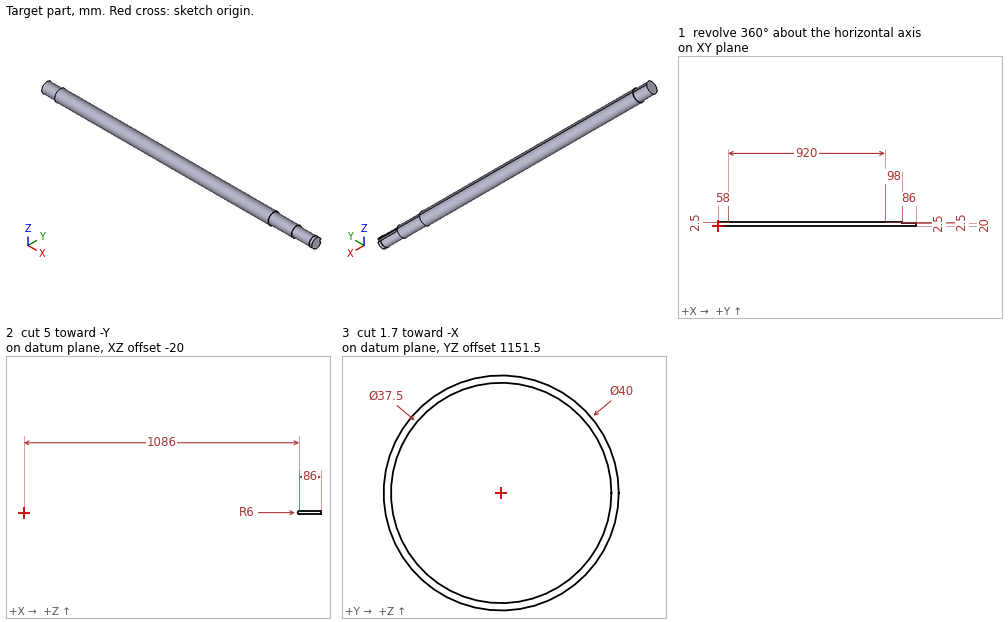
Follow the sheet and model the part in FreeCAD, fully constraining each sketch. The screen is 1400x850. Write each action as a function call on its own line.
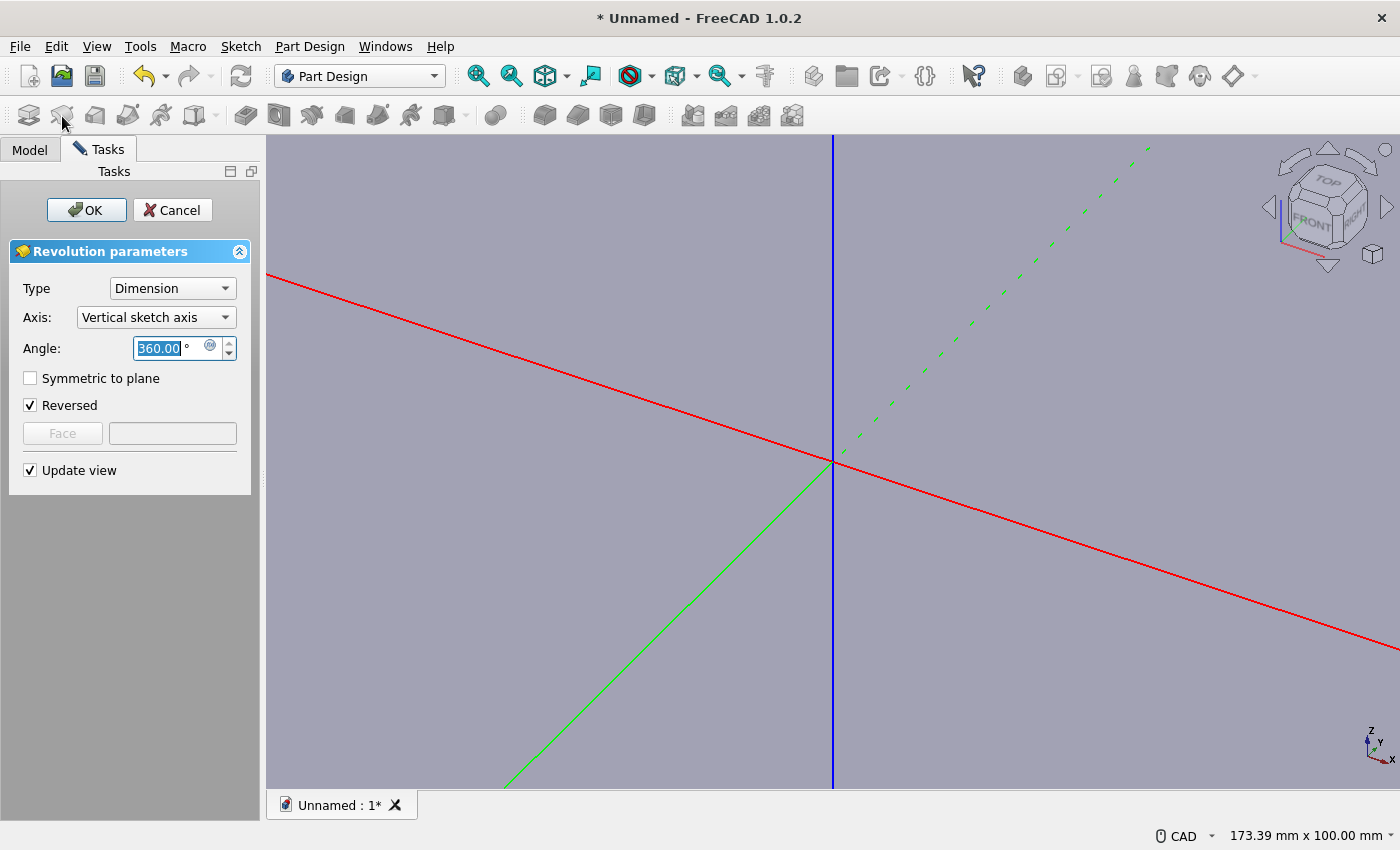
click(157, 318)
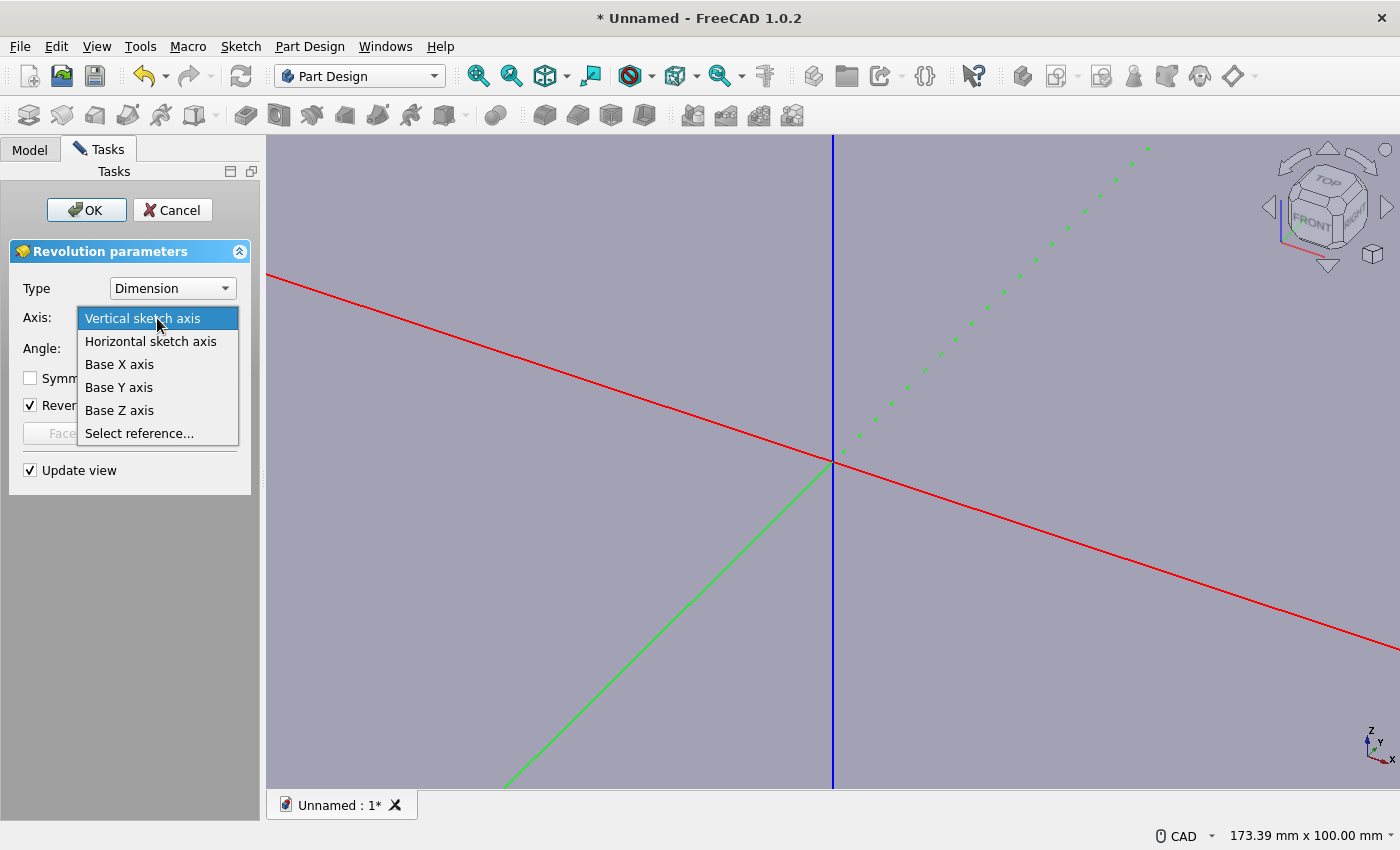
click(156, 342)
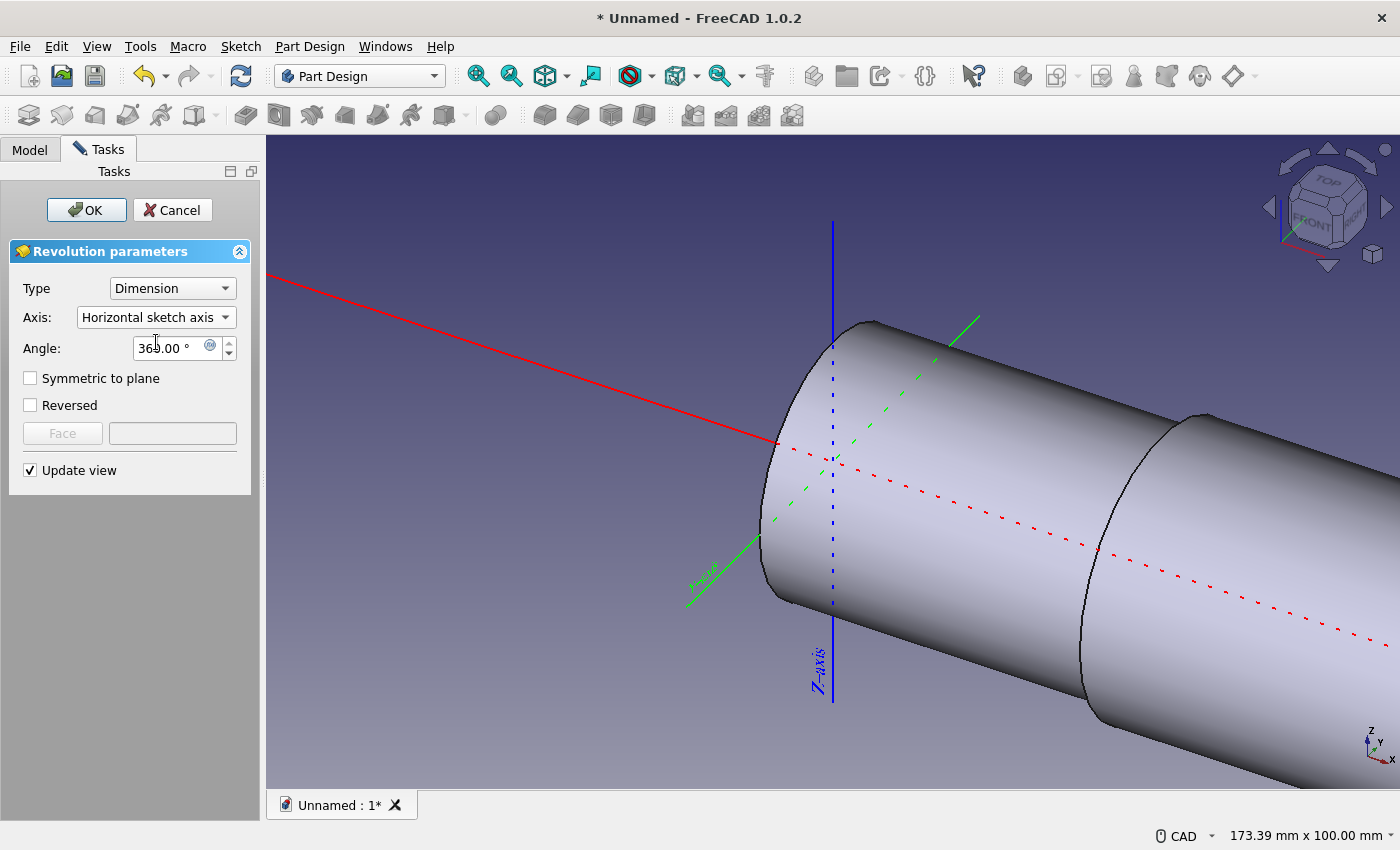
click(87, 210)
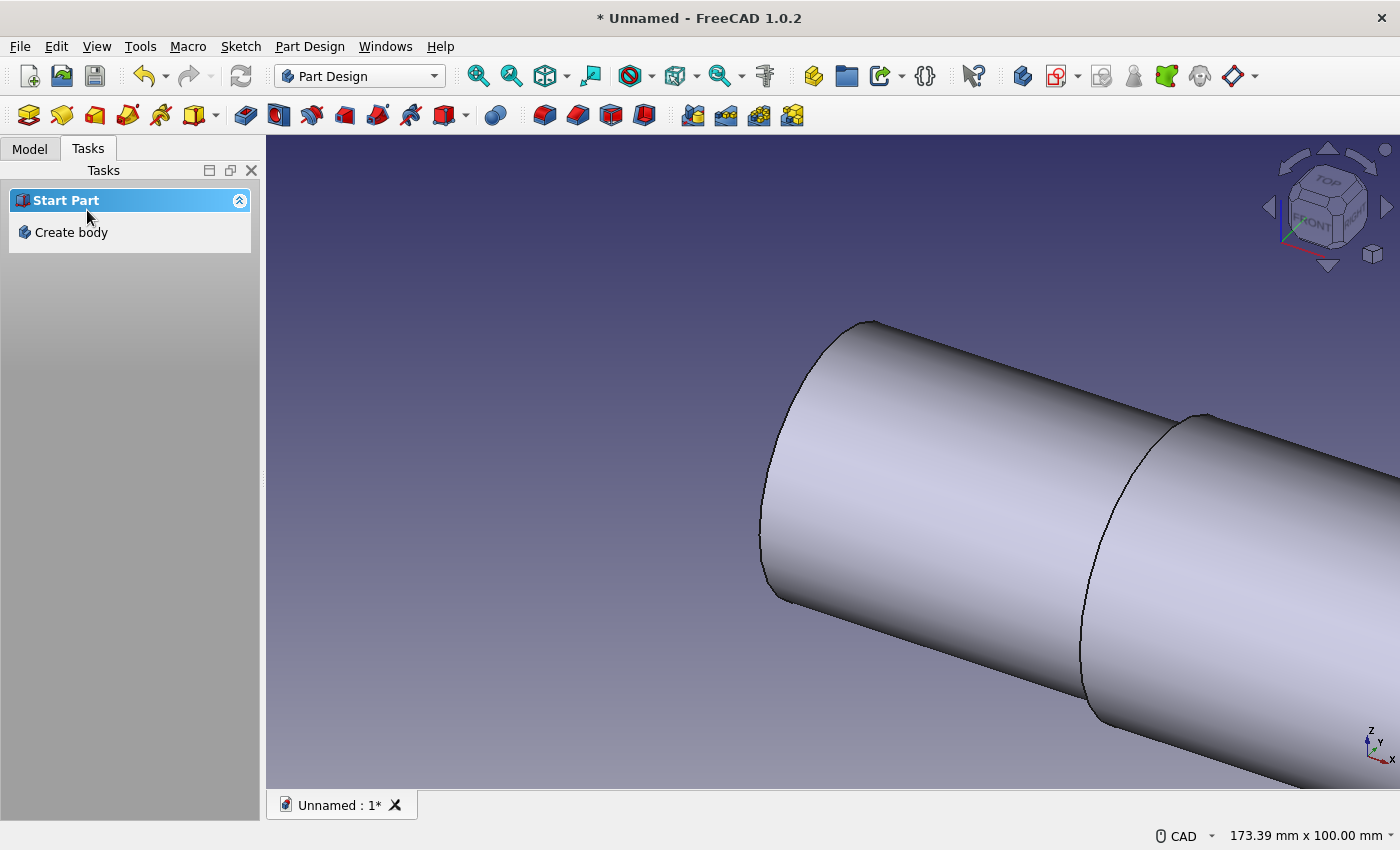
key(v)
key(f)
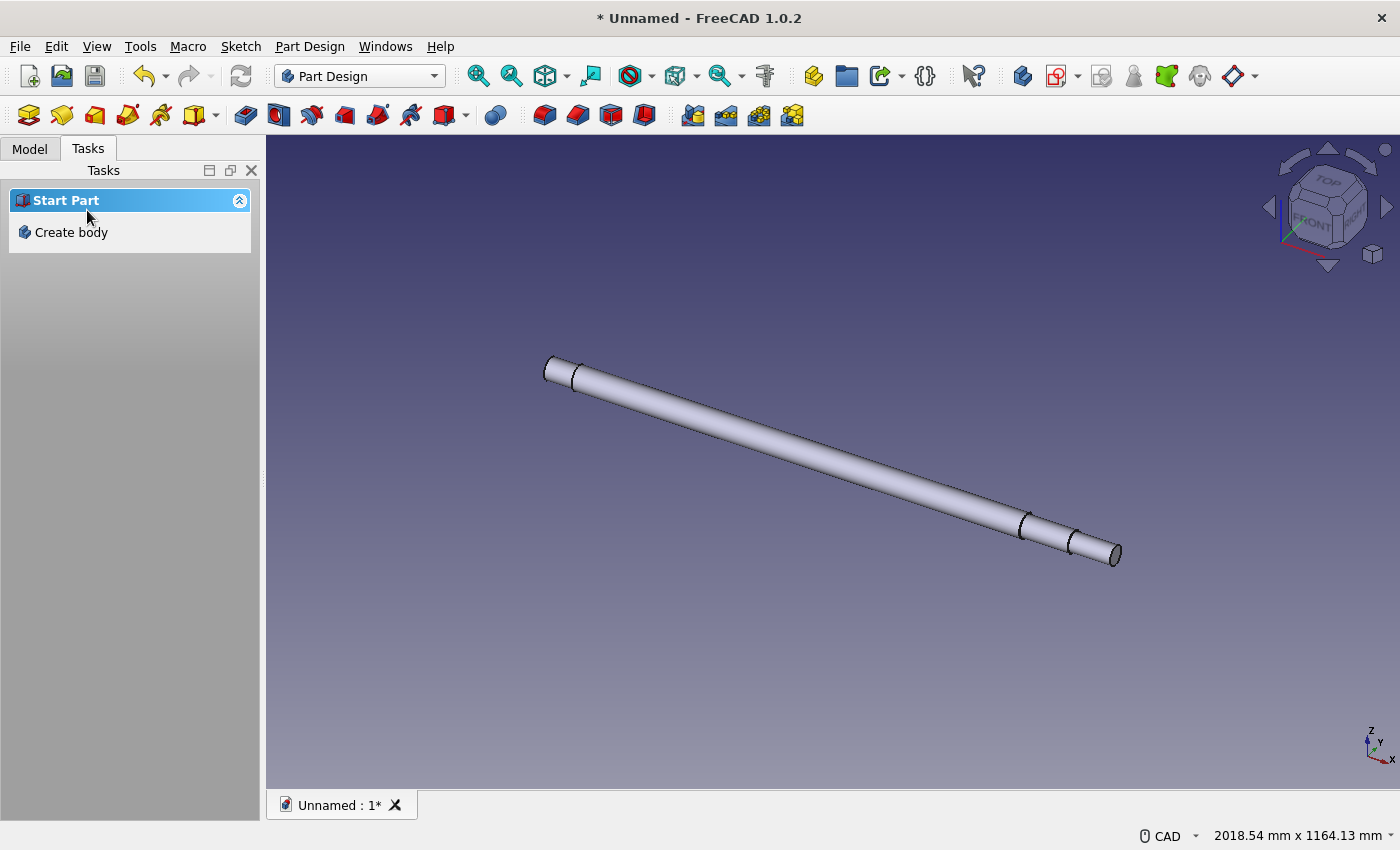
click(30, 148)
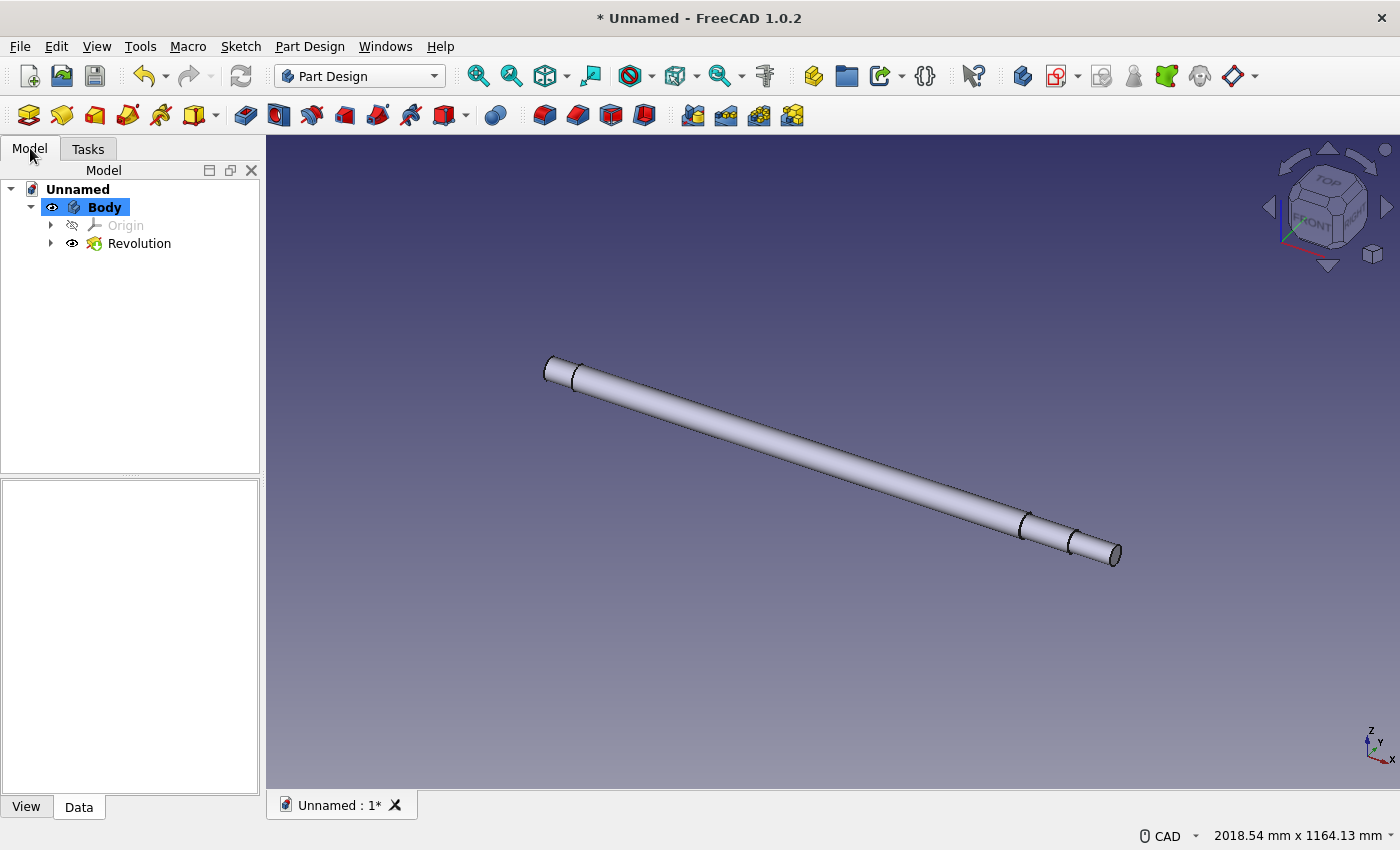
click(51, 225)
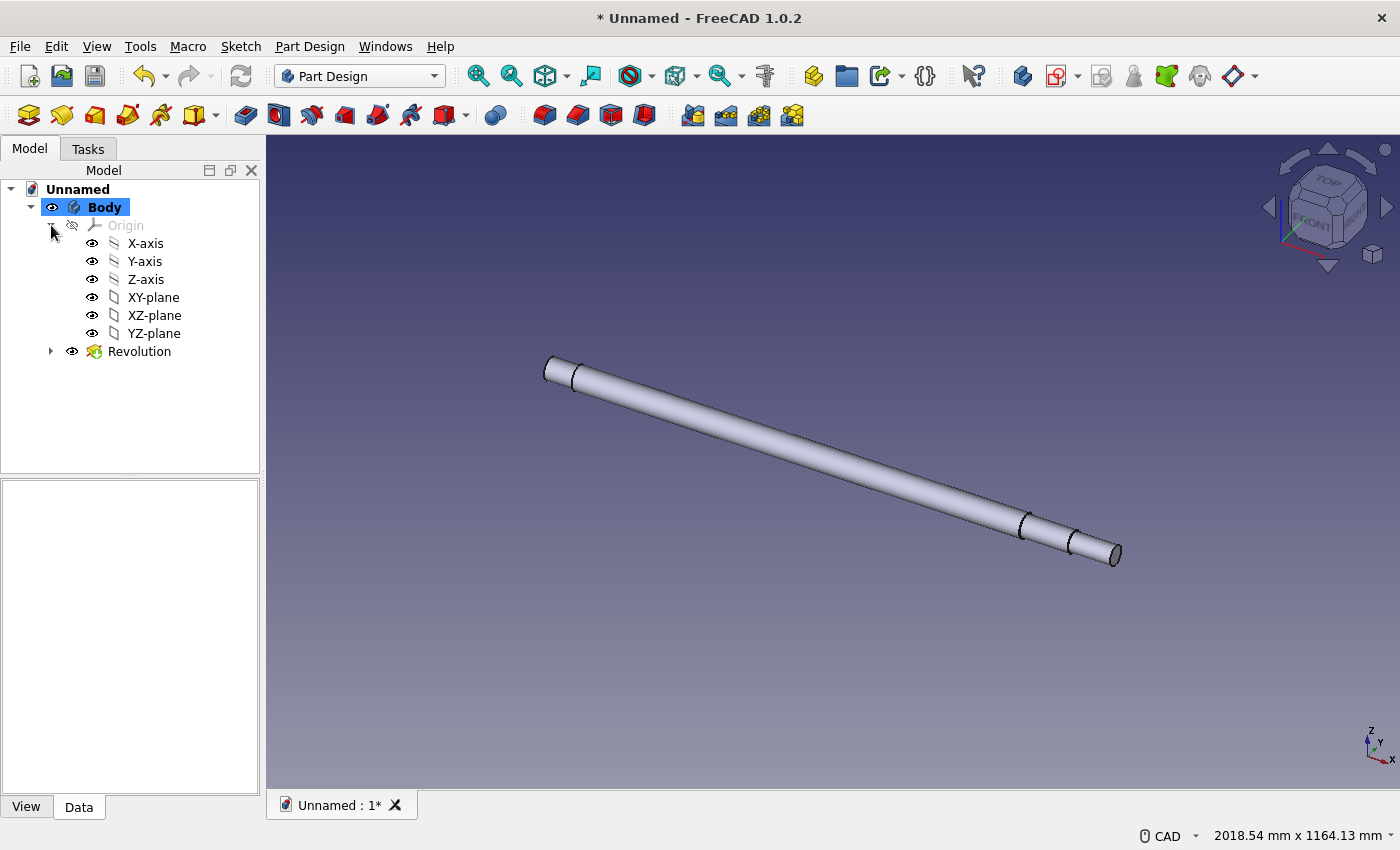
click(137, 315)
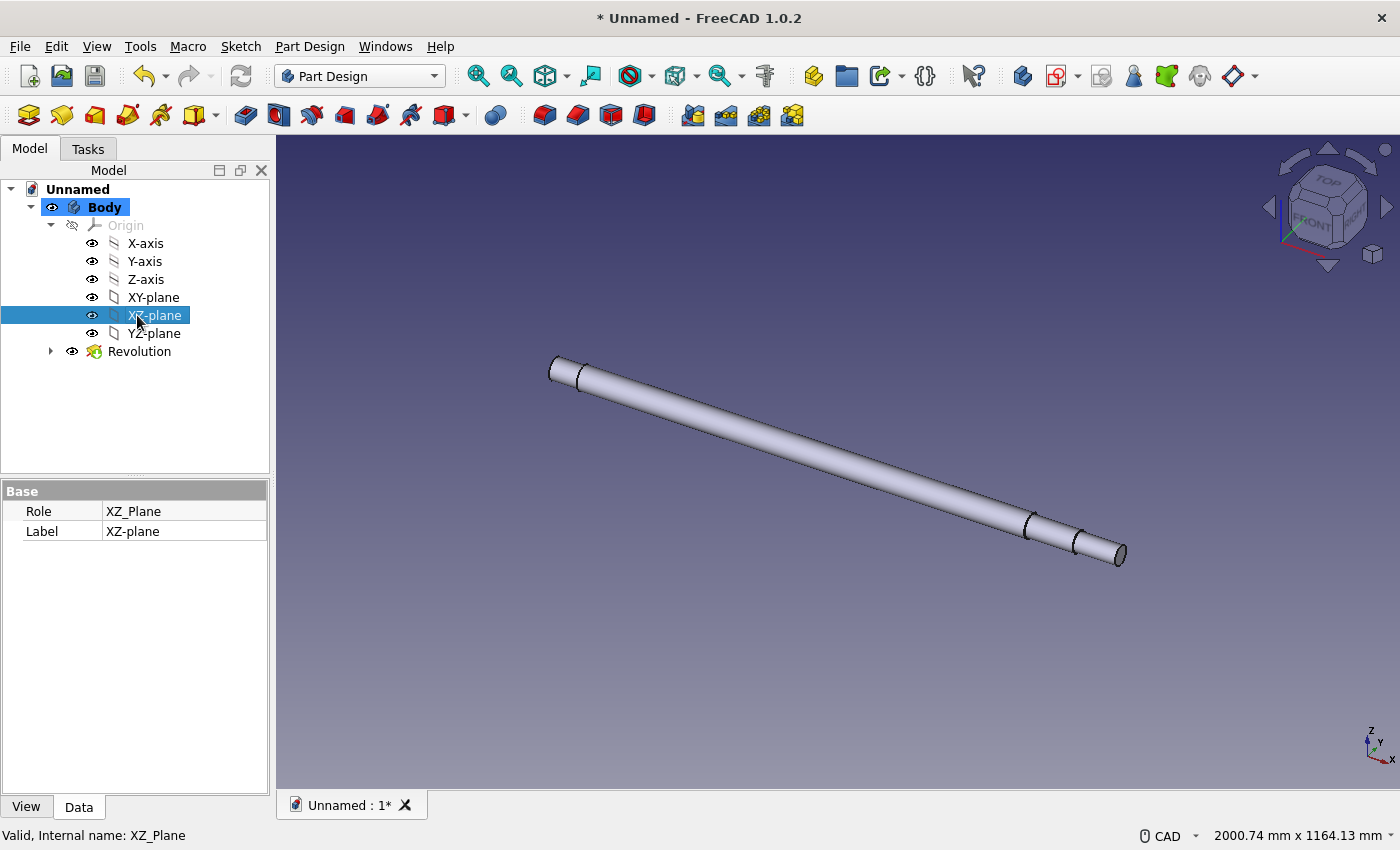
click(1232, 76)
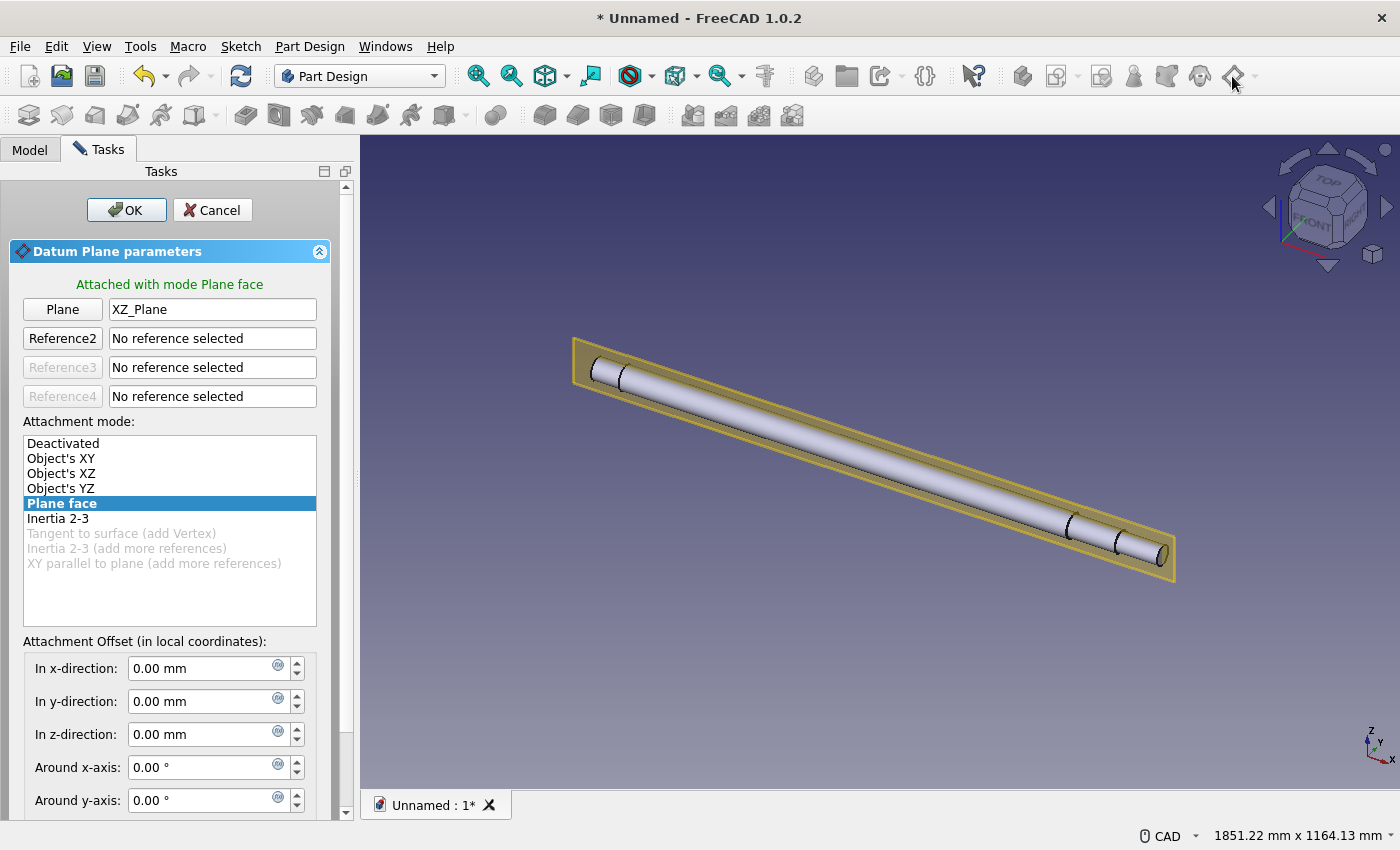
triple_click(210, 734)